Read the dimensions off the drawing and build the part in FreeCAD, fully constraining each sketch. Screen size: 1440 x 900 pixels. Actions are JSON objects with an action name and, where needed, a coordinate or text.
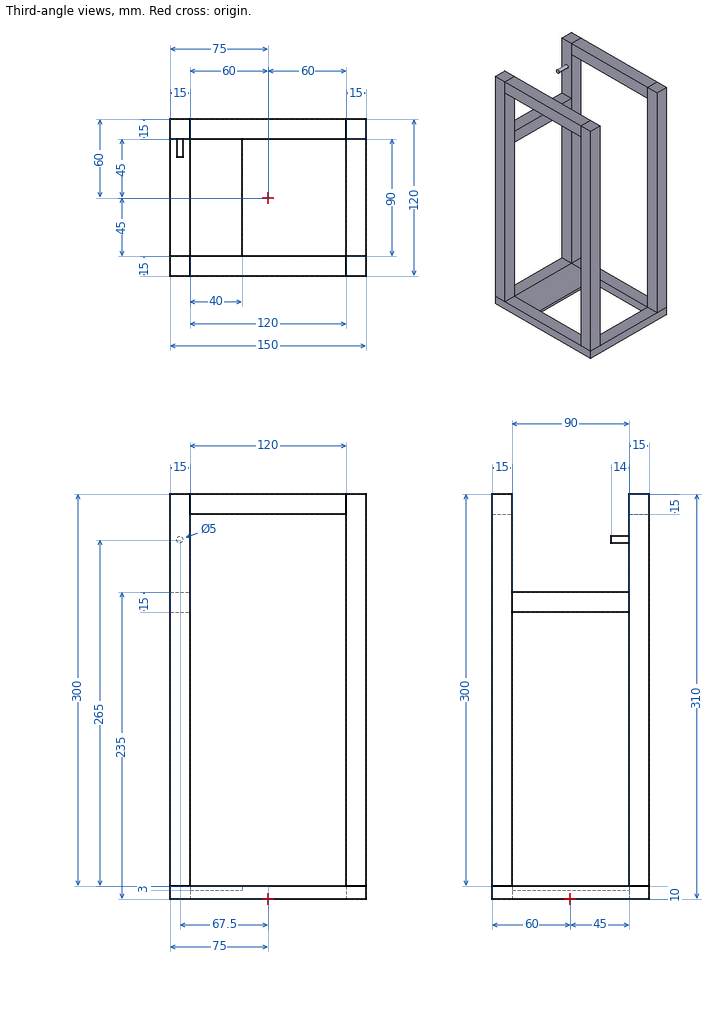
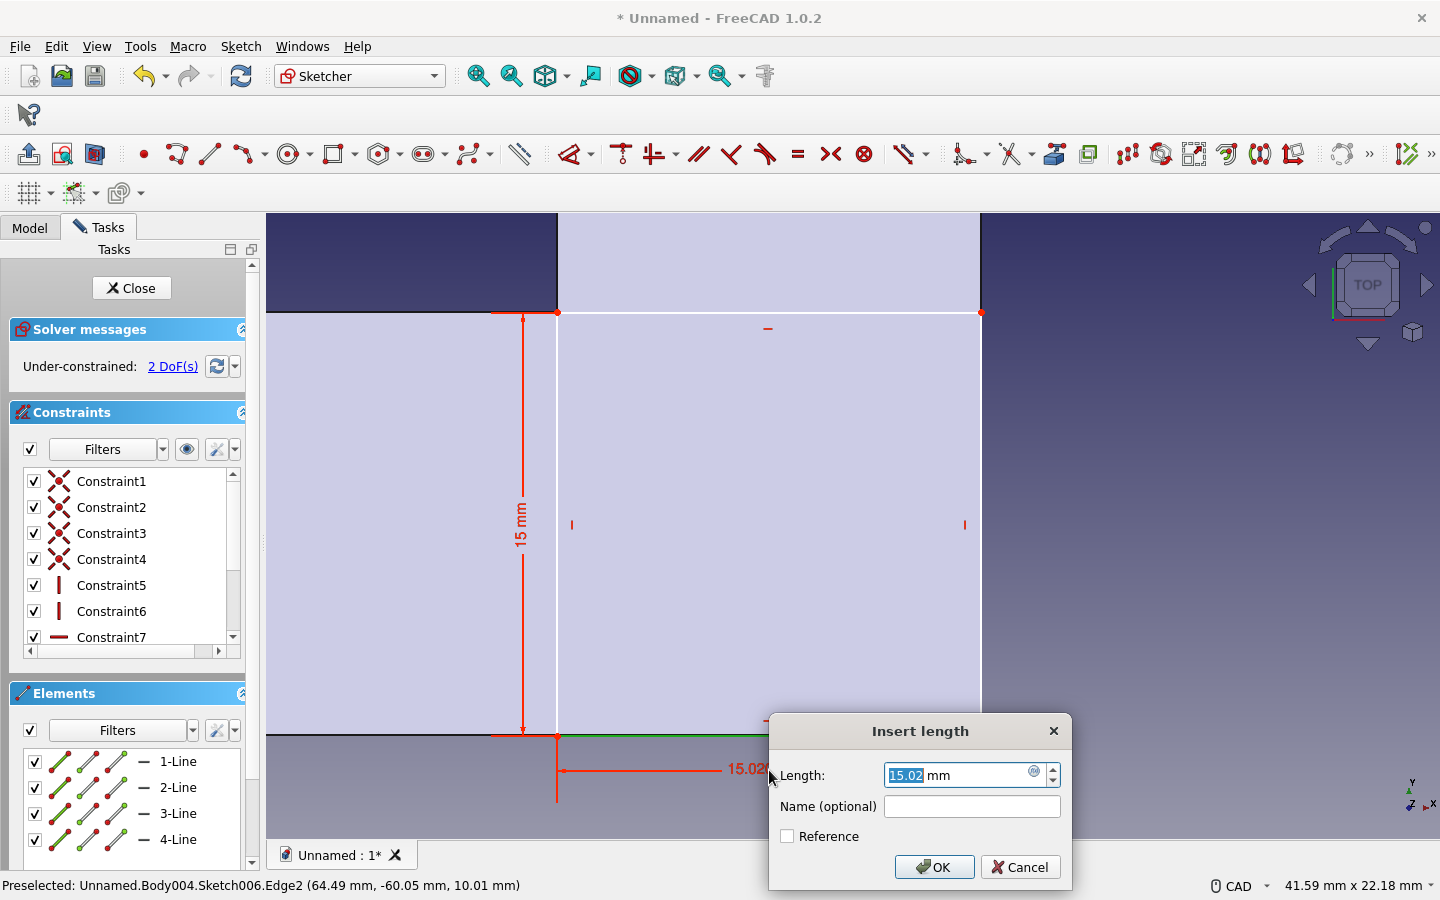
{"action": "type", "text": "15"}
{"action": "key", "text": "Return"}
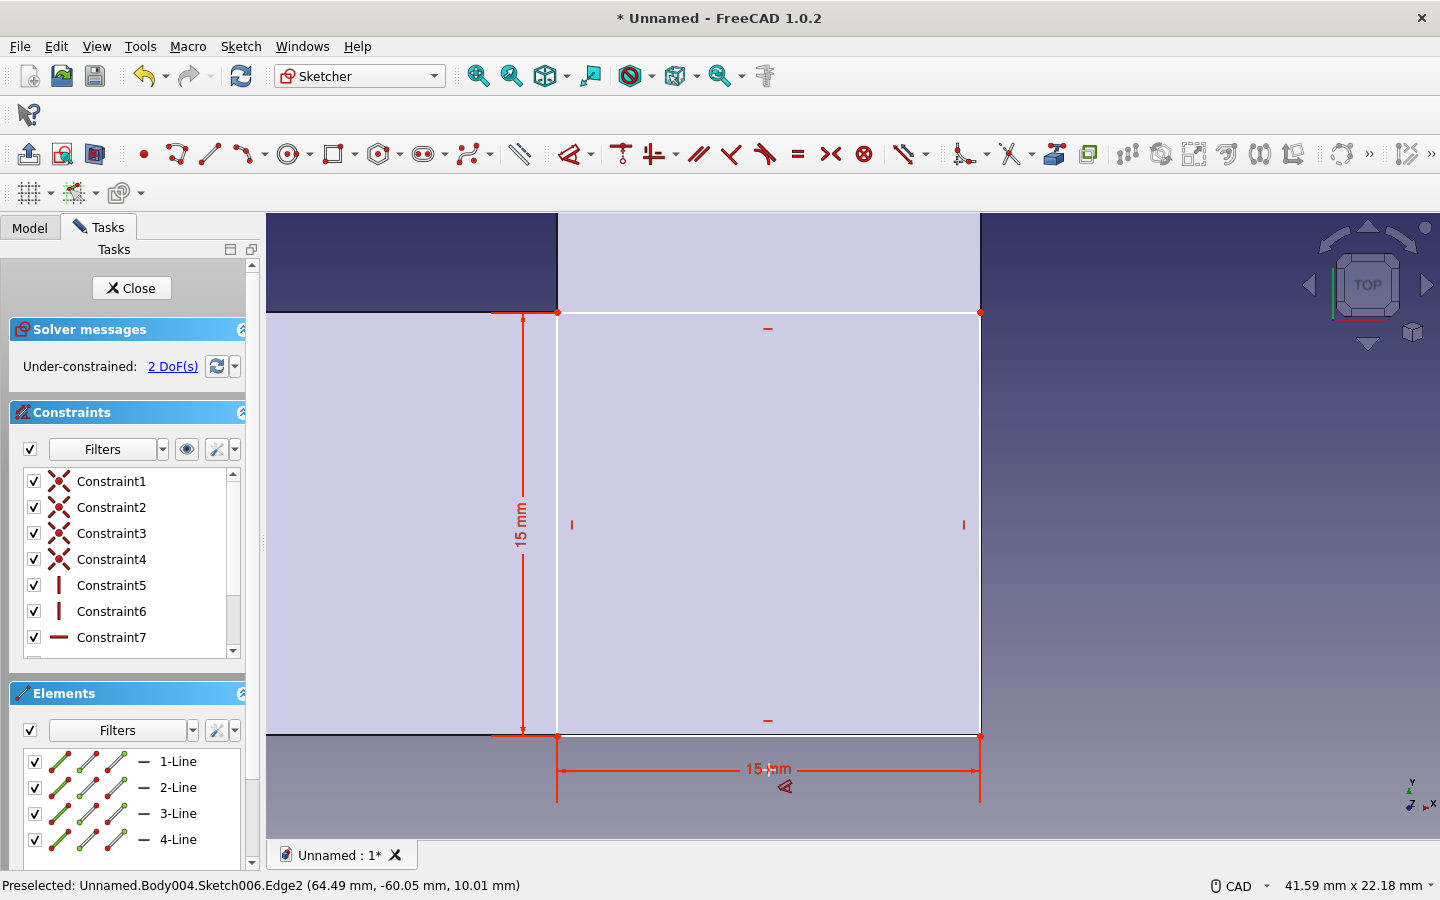
{"action": "left_click", "coordinate": [557, 313]}
{"action": "left_click", "coordinate": [426, 347]}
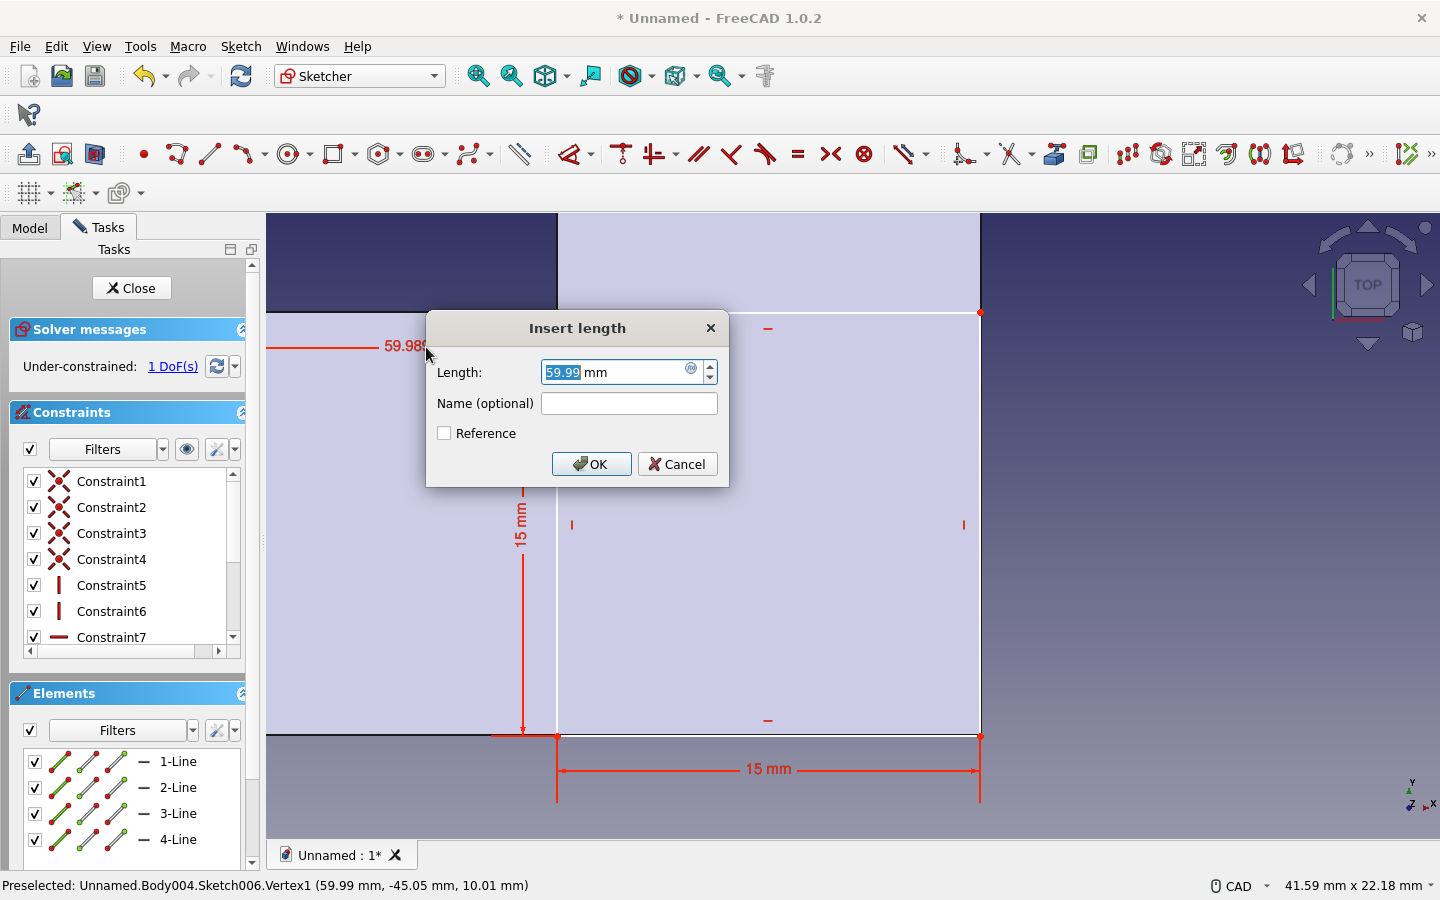
{"action": "type", "text": "60"}
{"action": "key", "text": "Return"}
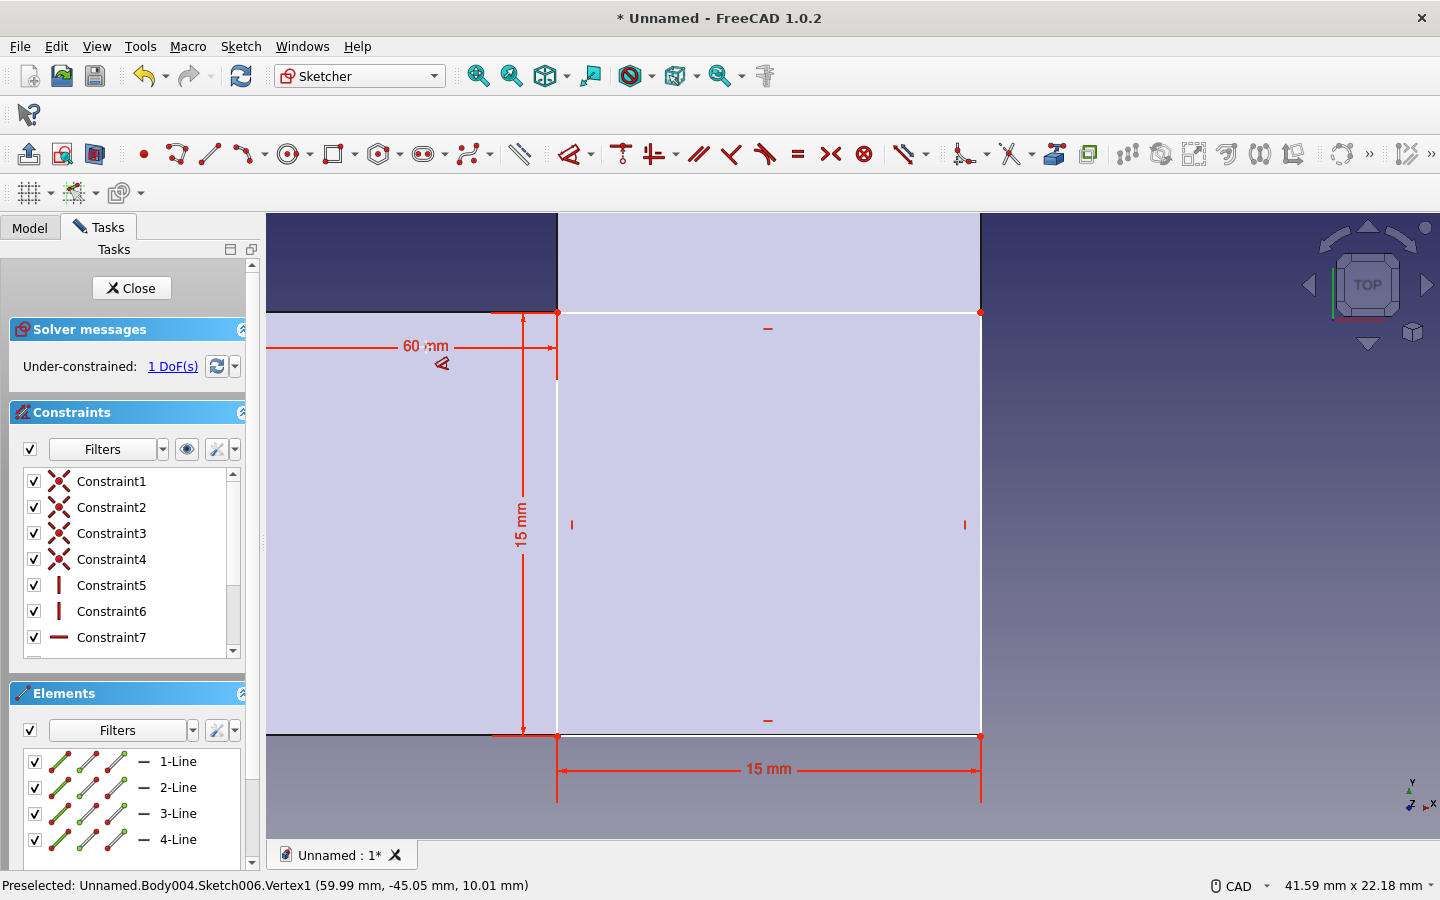
{"action": "left_click", "coordinate": [557, 313]}
{"action": "left_click", "coordinate": [591, 277]}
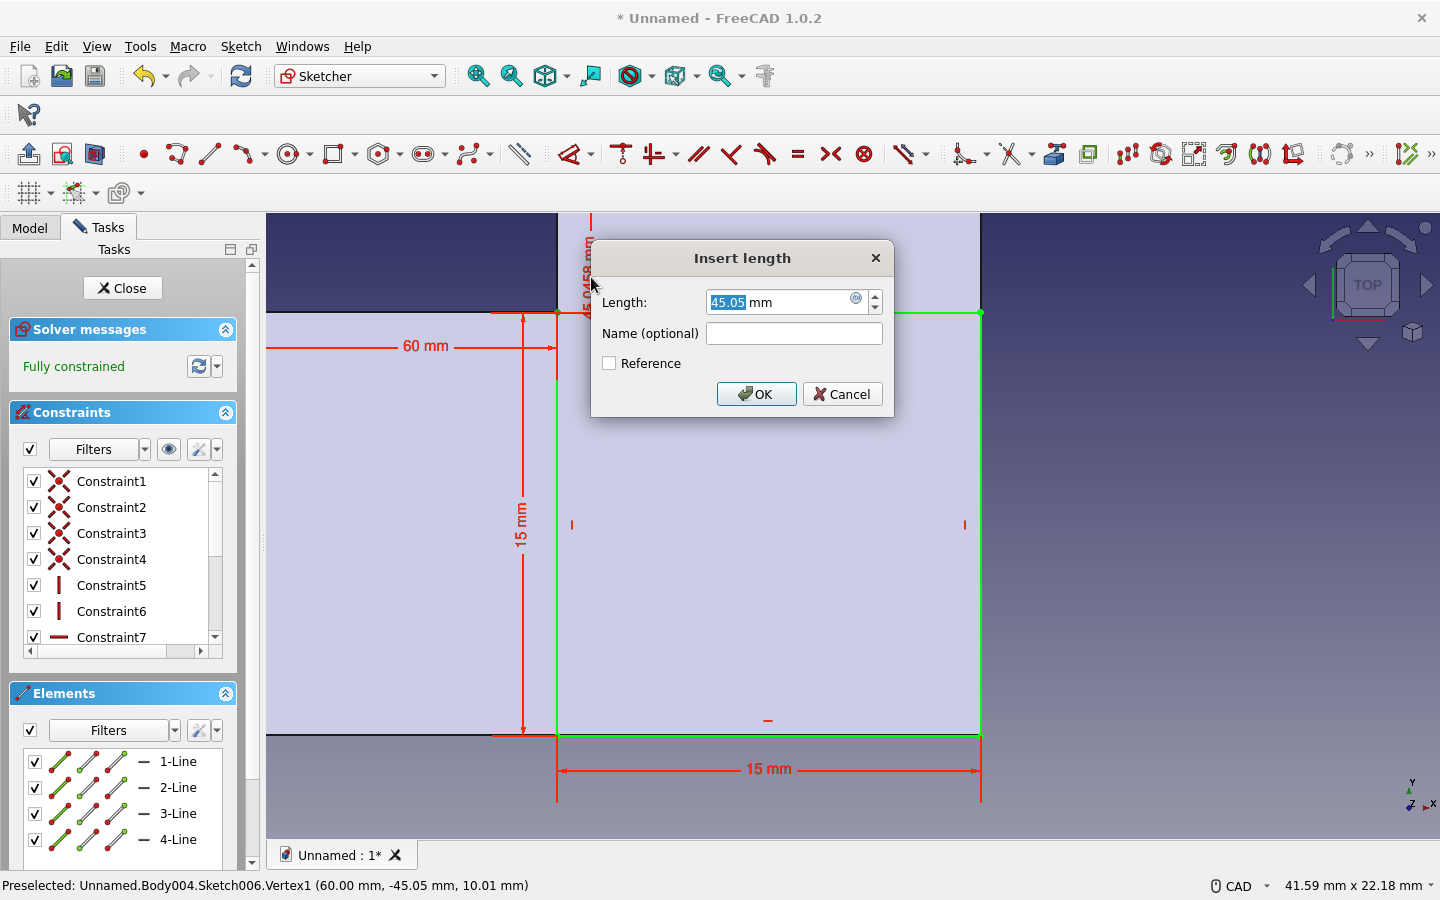
{"action": "type", "text": "45"}
{"action": "key", "text": "Return"}
{"action": "key", "text": "Escape"}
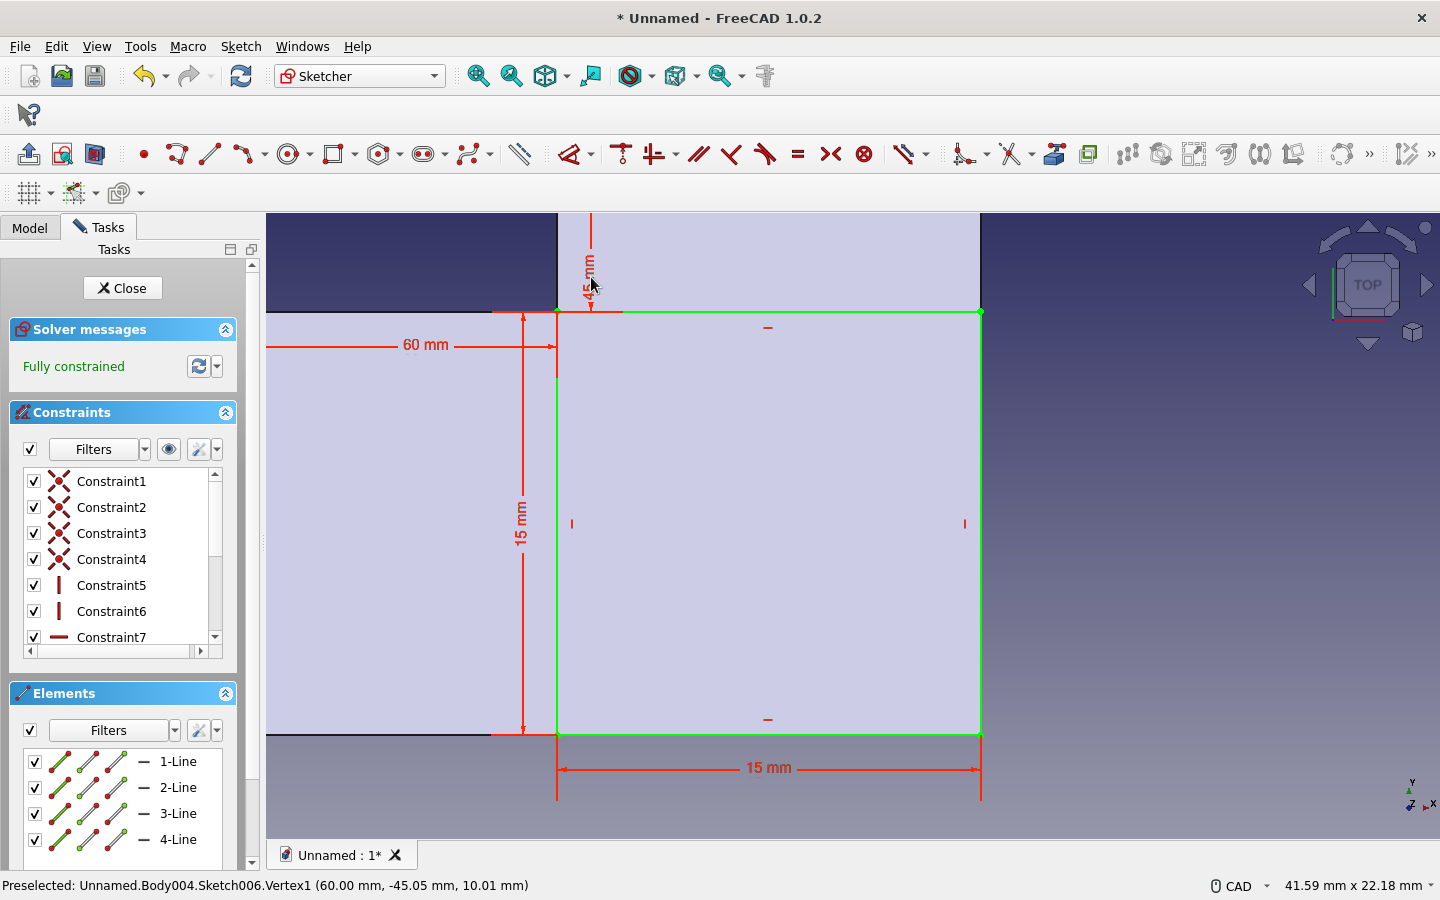
{"action": "left_click", "coordinate": [123, 288]}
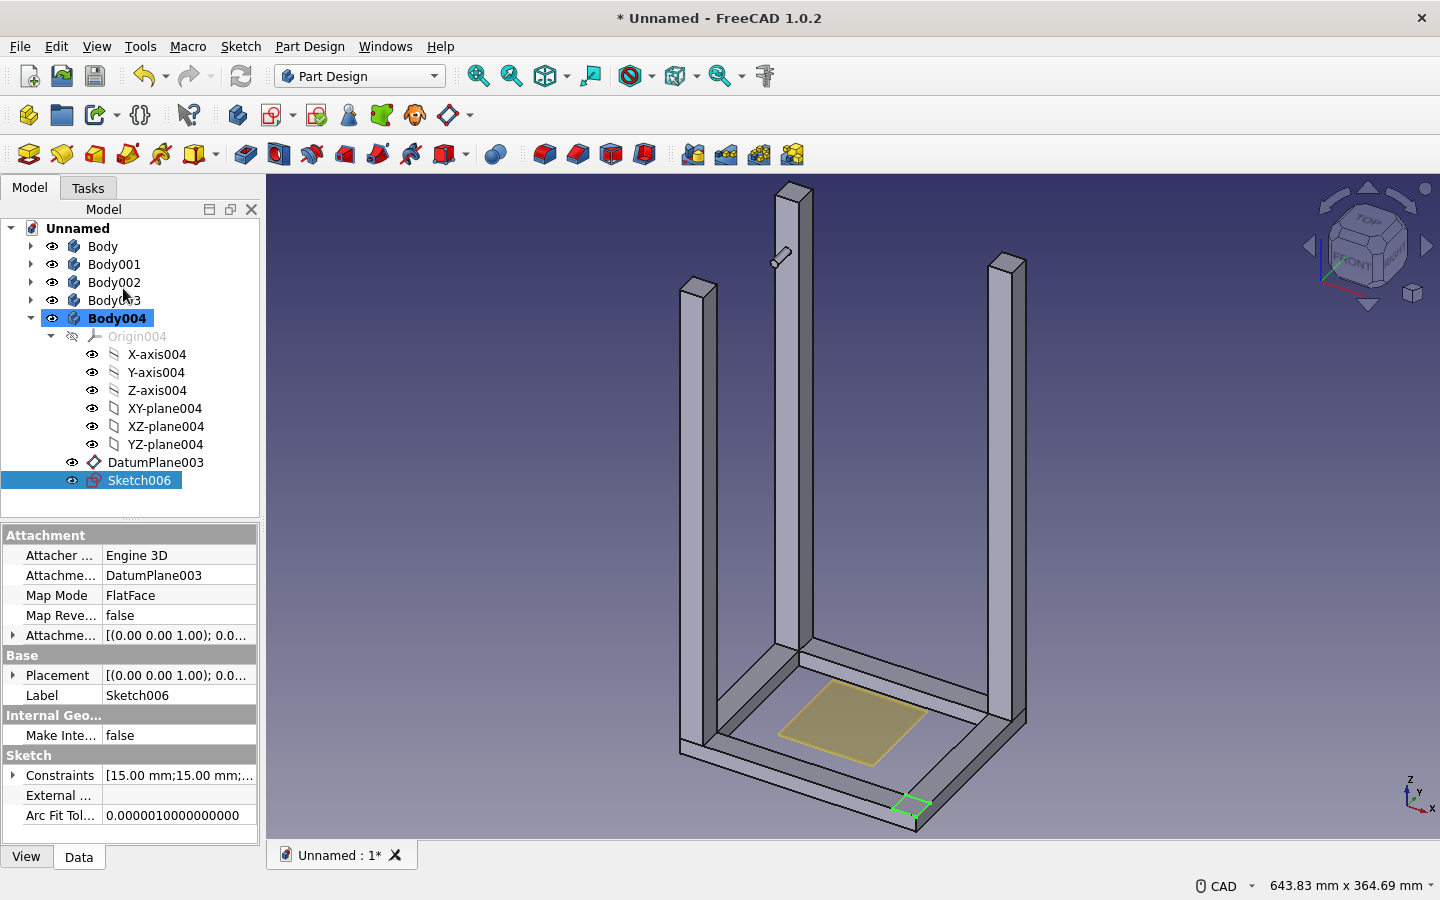
{"action": "left_click", "coordinate": [29, 154]}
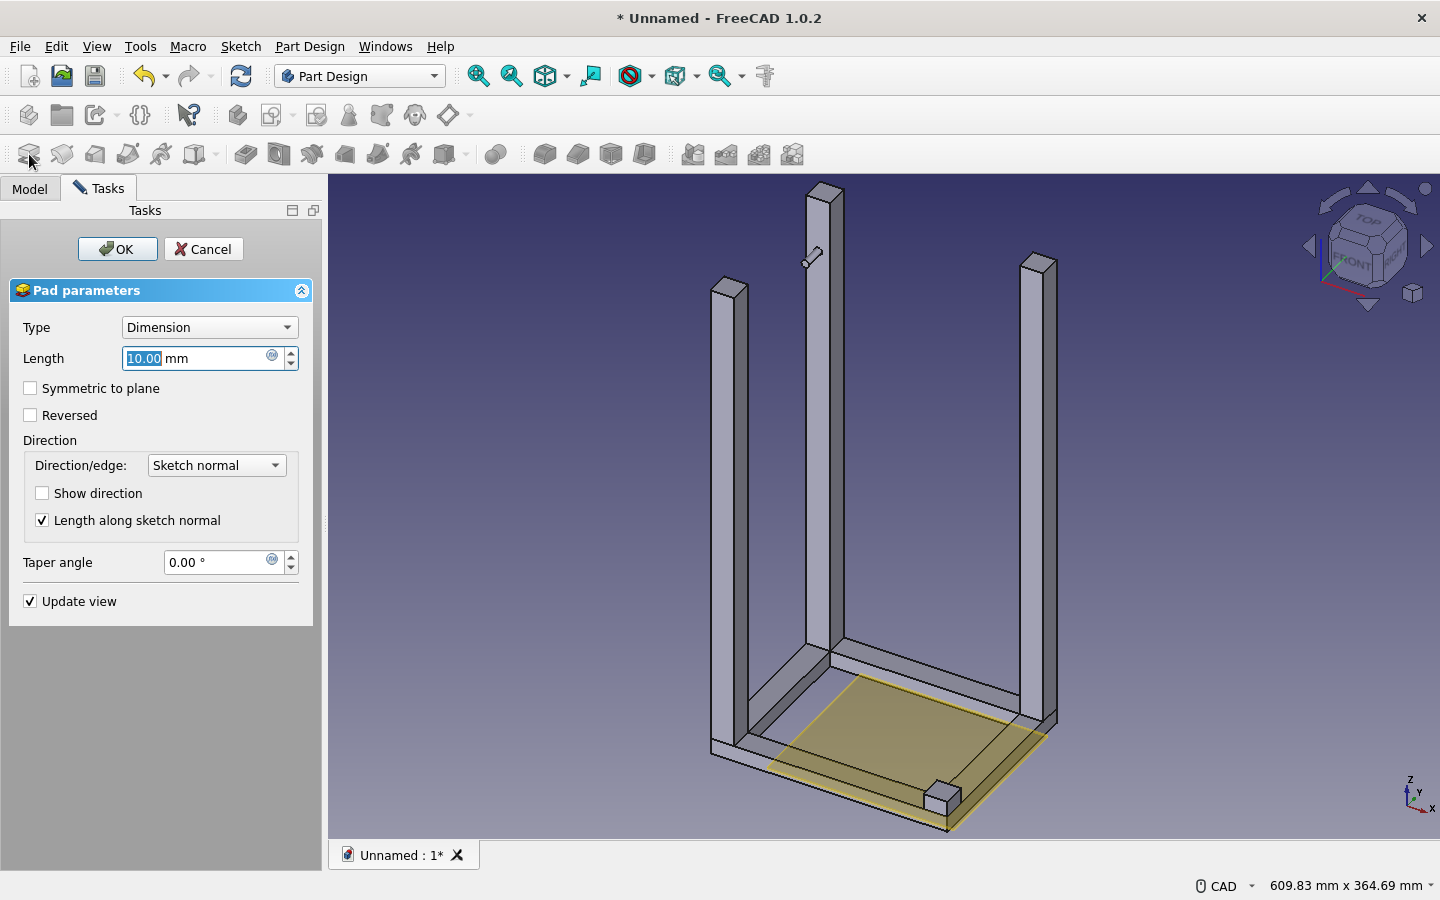
{"action": "type", "text": "300"}
{"action": "key", "text": "Tab"}